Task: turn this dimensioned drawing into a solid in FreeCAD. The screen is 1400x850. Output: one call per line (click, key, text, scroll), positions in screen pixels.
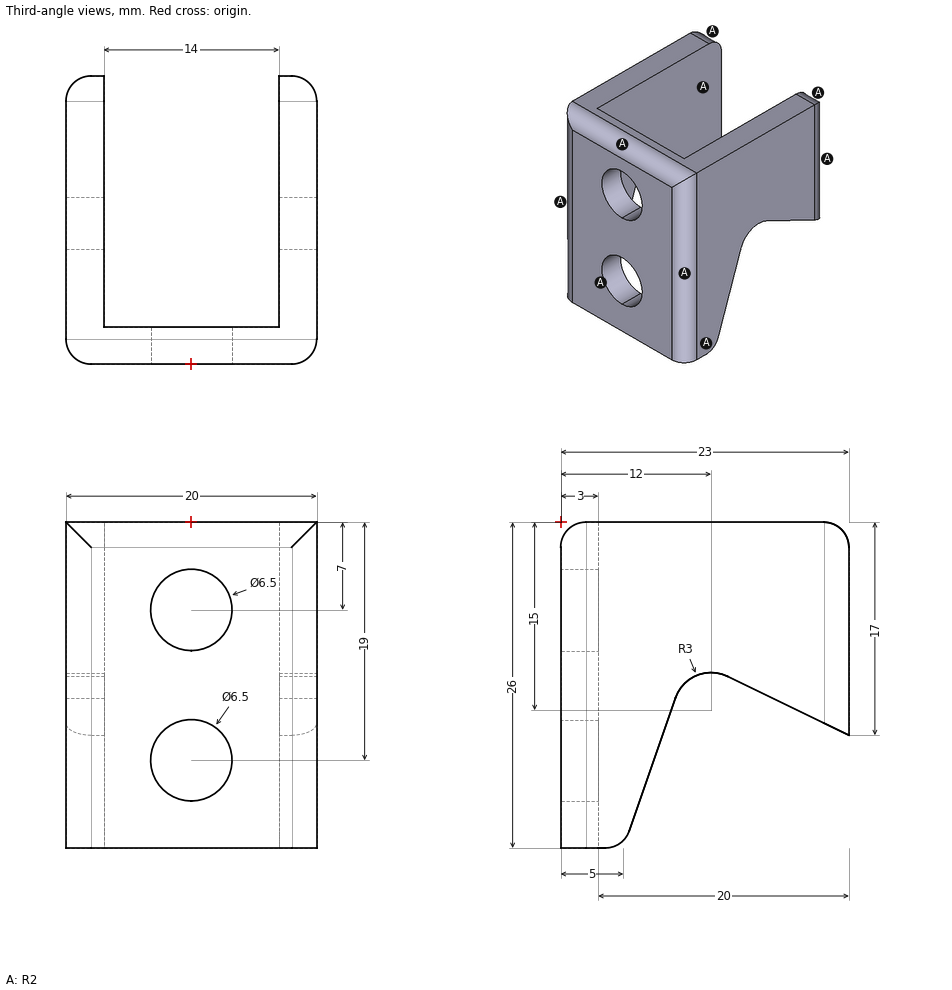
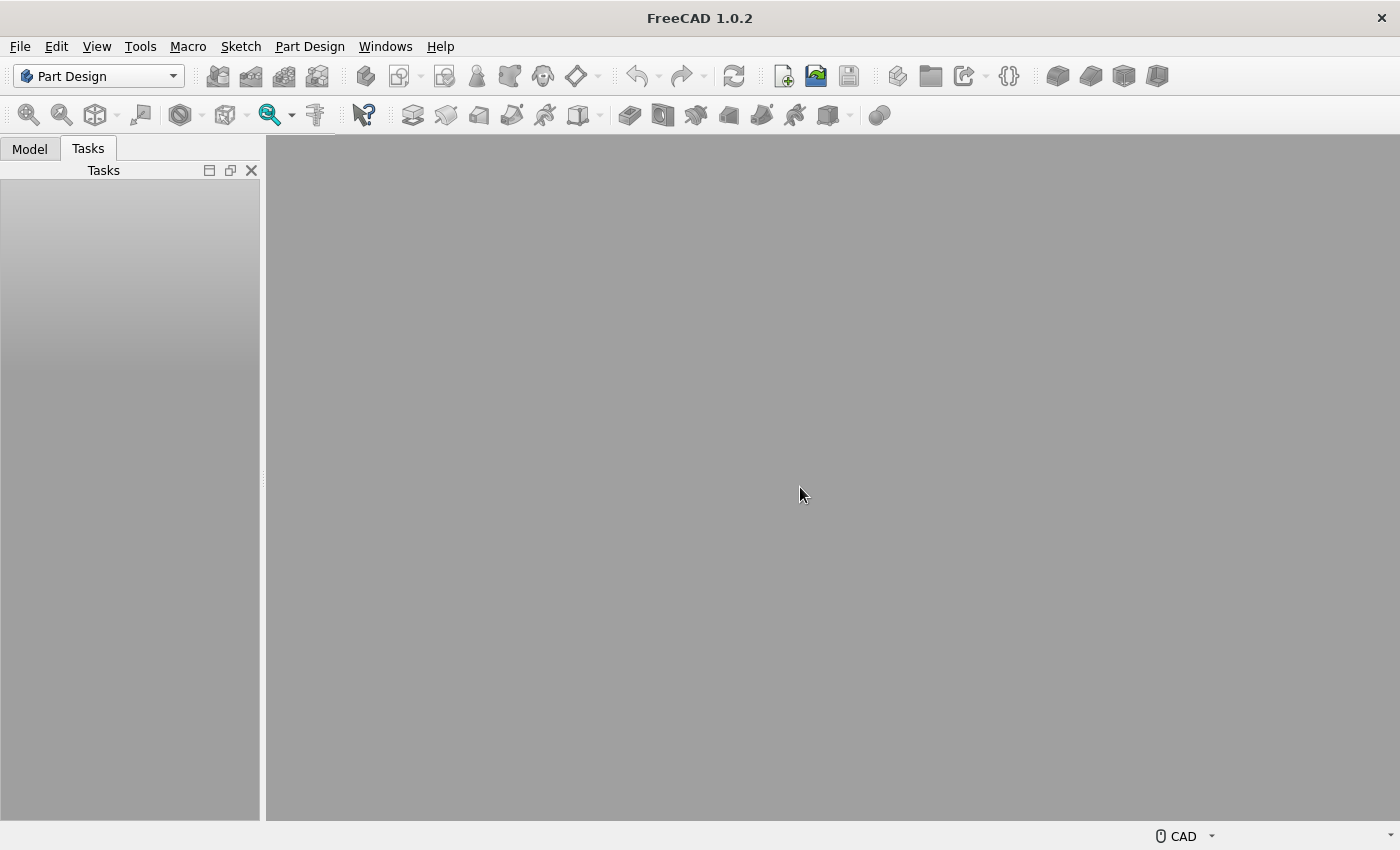
click(783, 76)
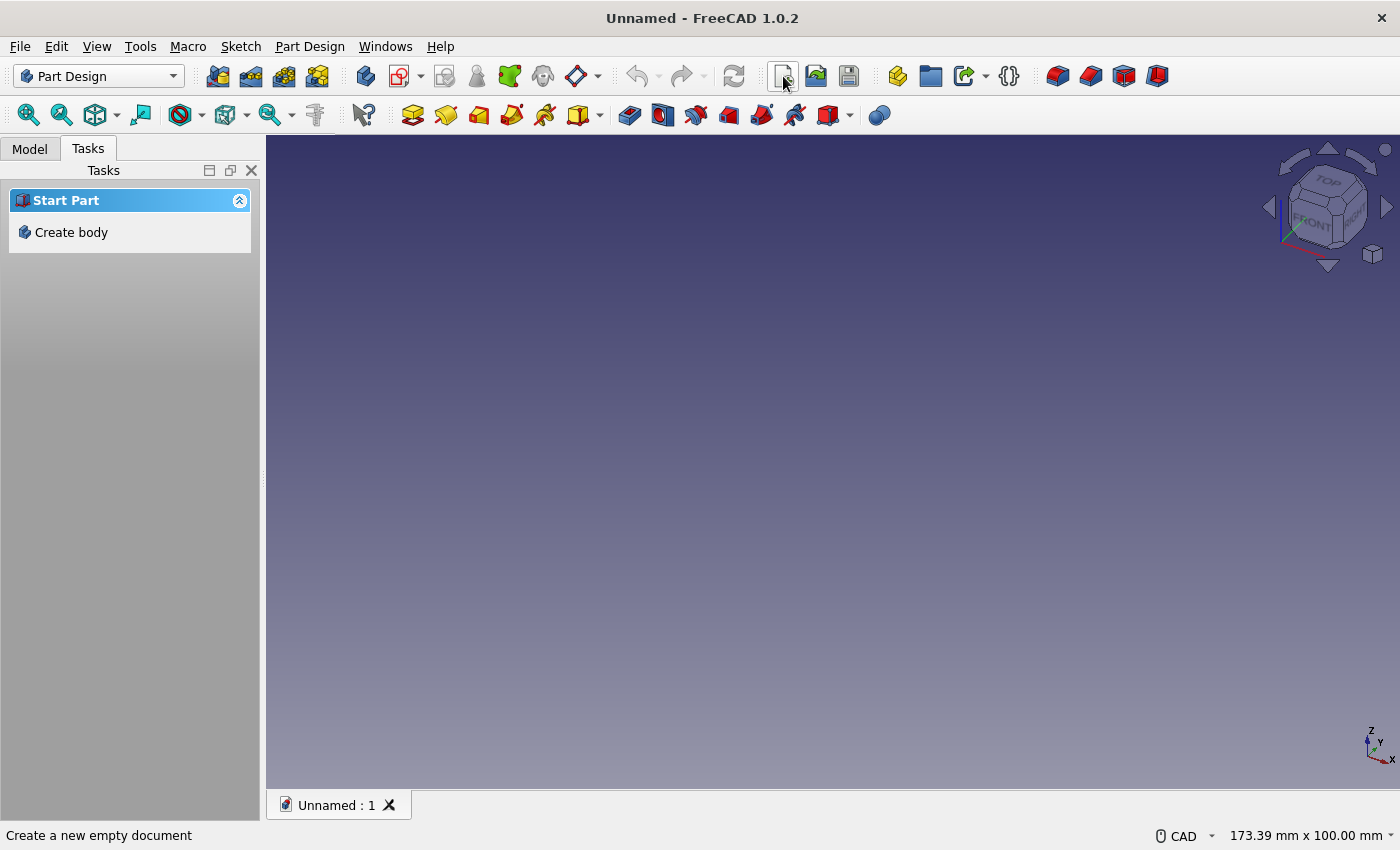
click(398, 76)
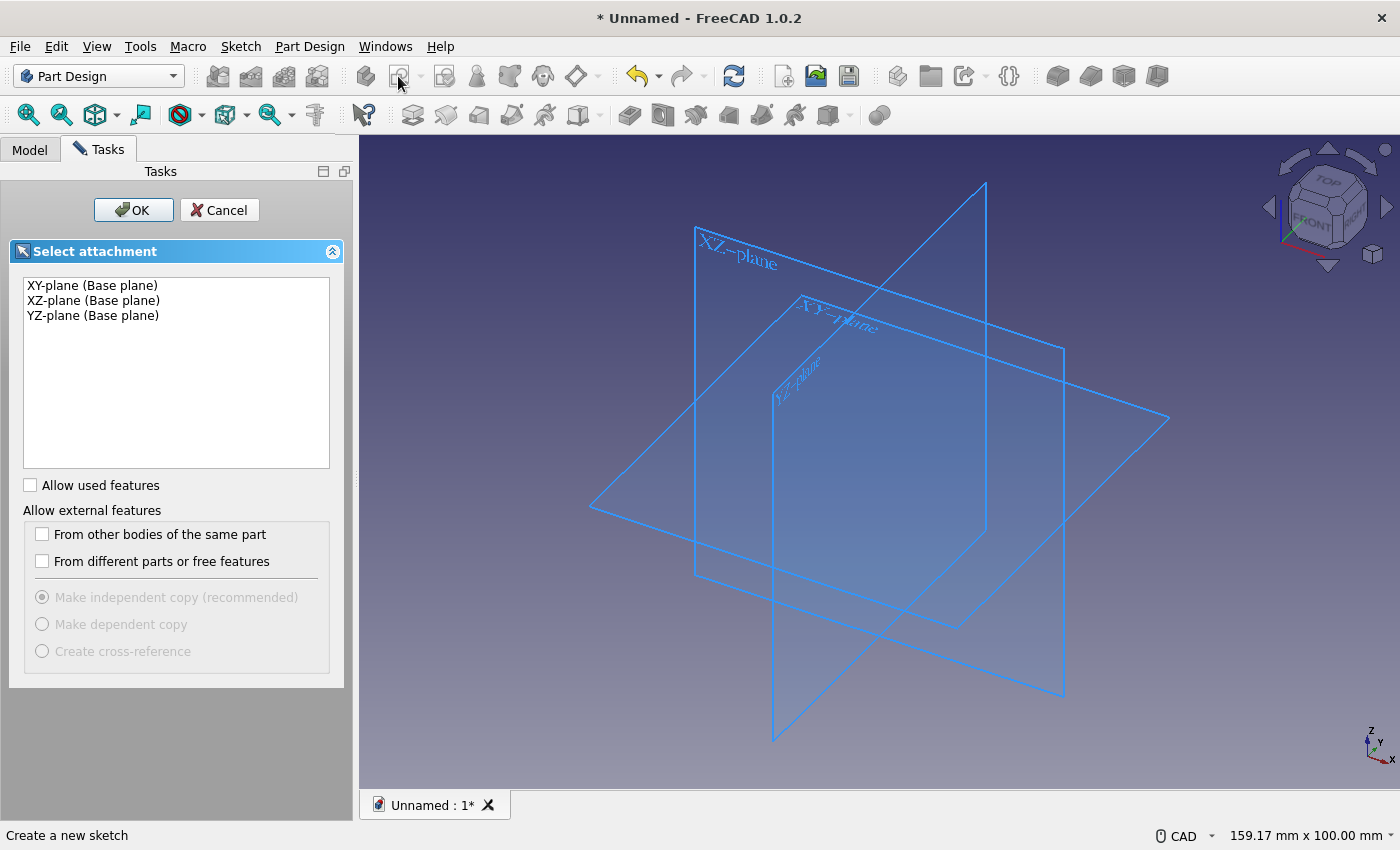
click(84, 316)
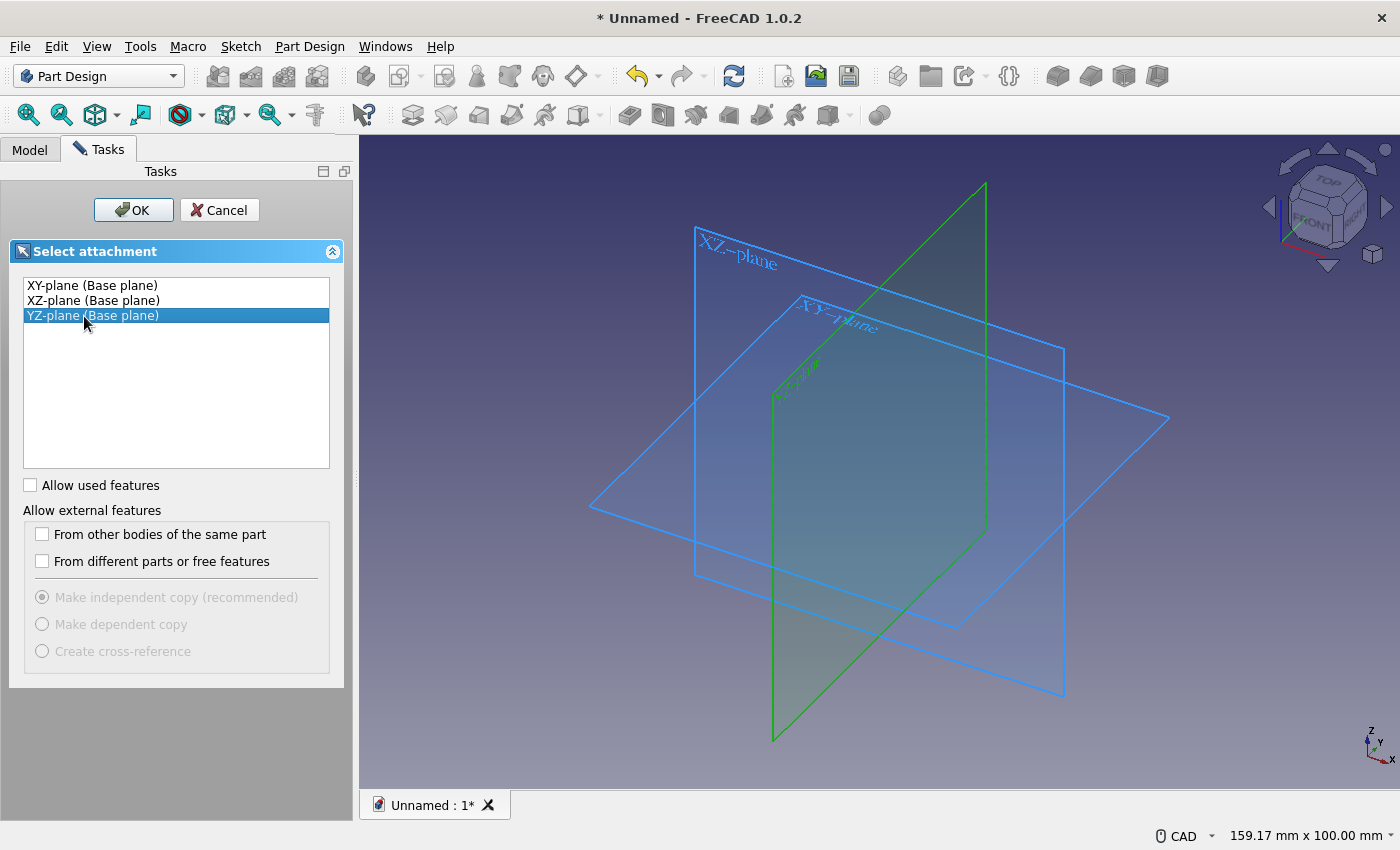
click(134, 210)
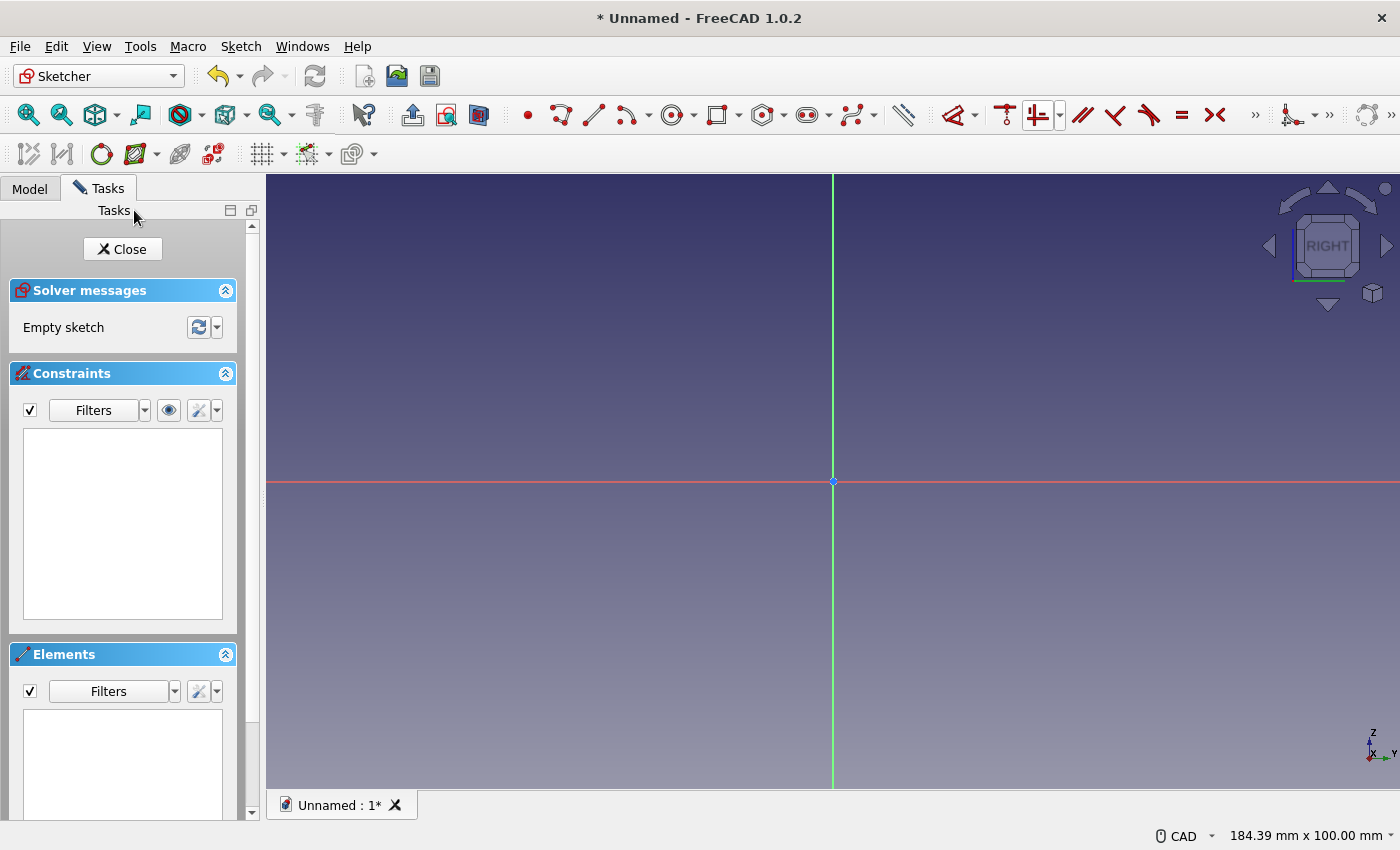
scroll(985, 608, up, 5)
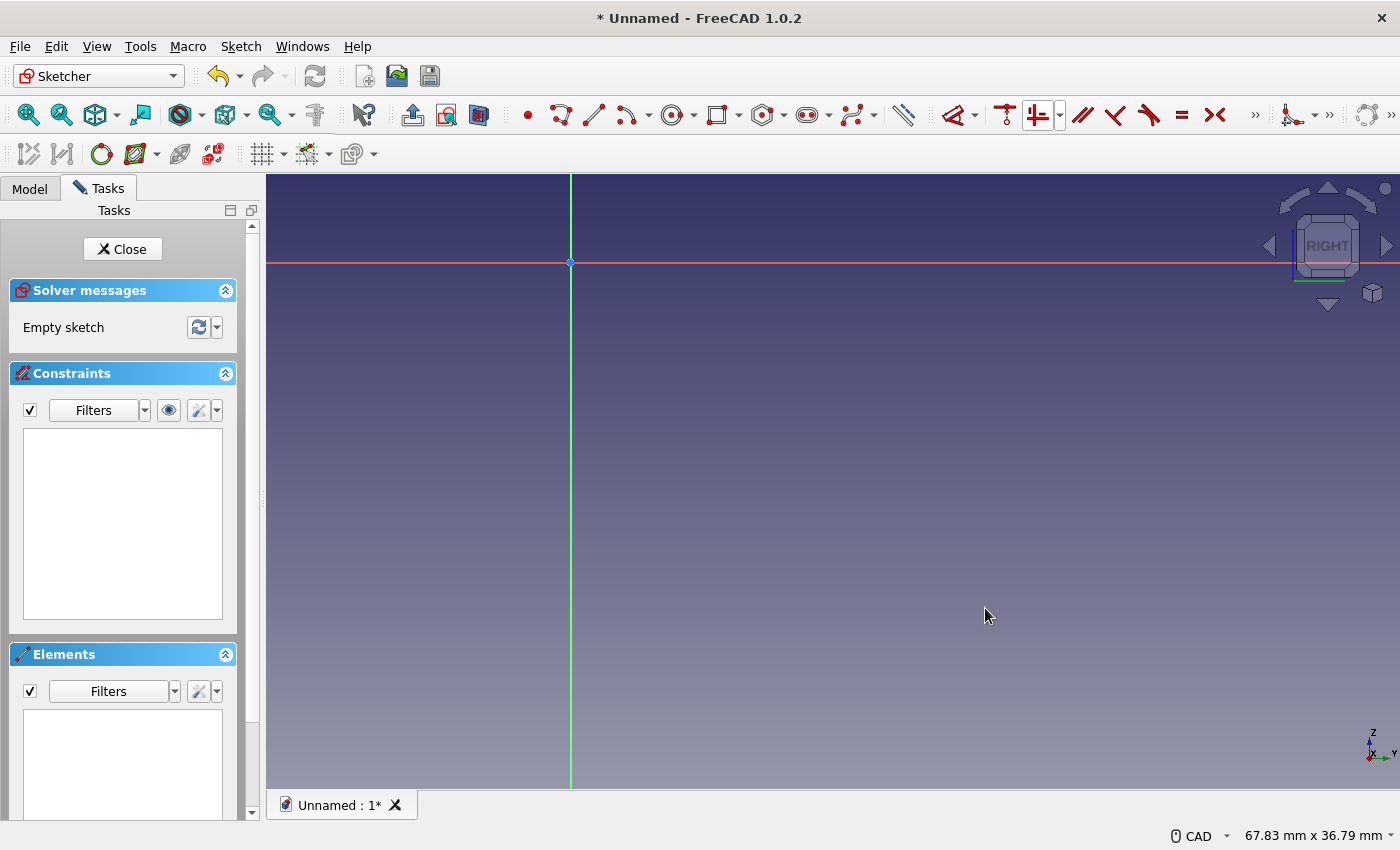
click(561, 116)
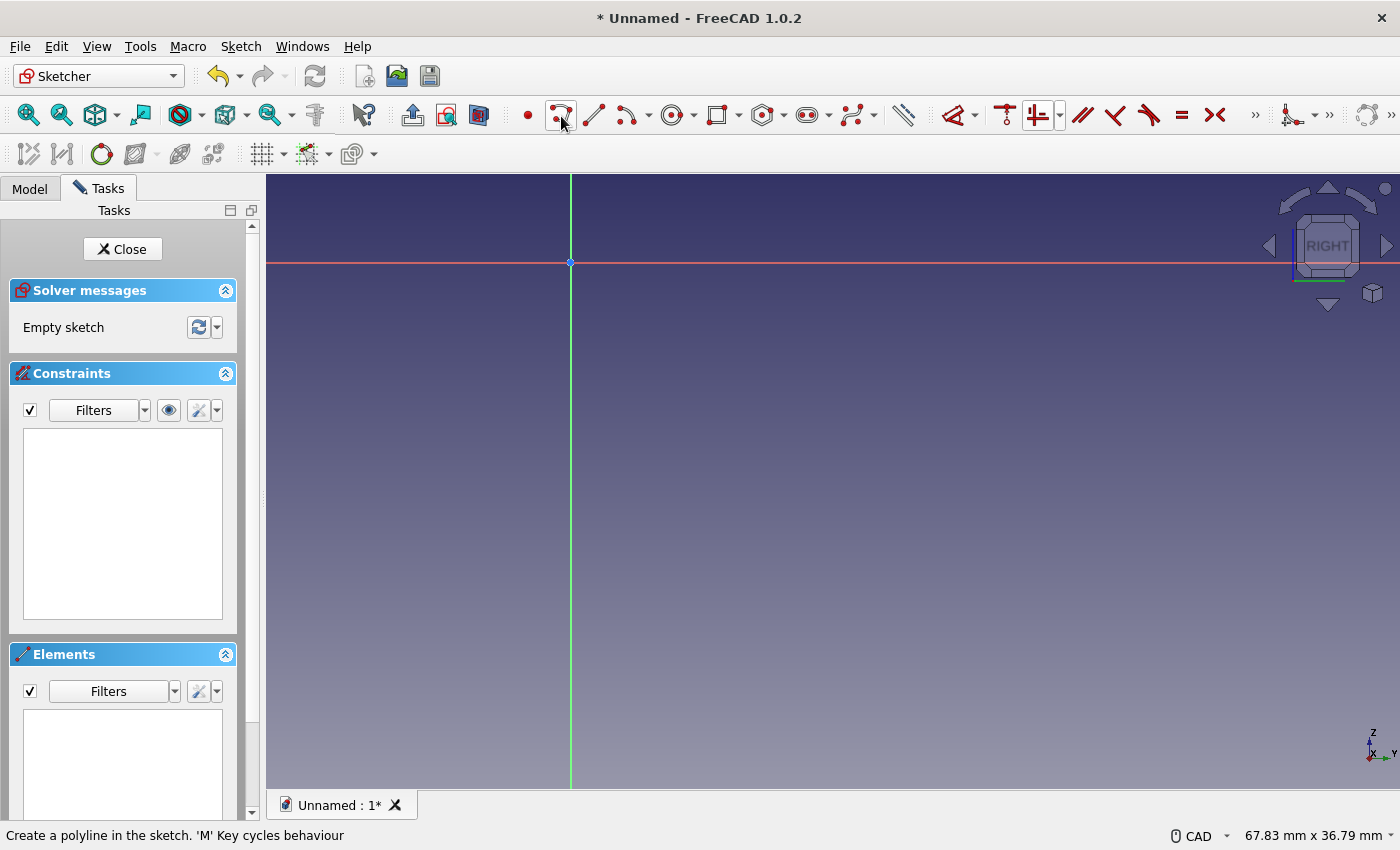
click(793, 469)
click(955, 547)
click(955, 263)
click(571, 263)
click(580, 698)
click(654, 698)
click(724, 497)
right_click(724, 497)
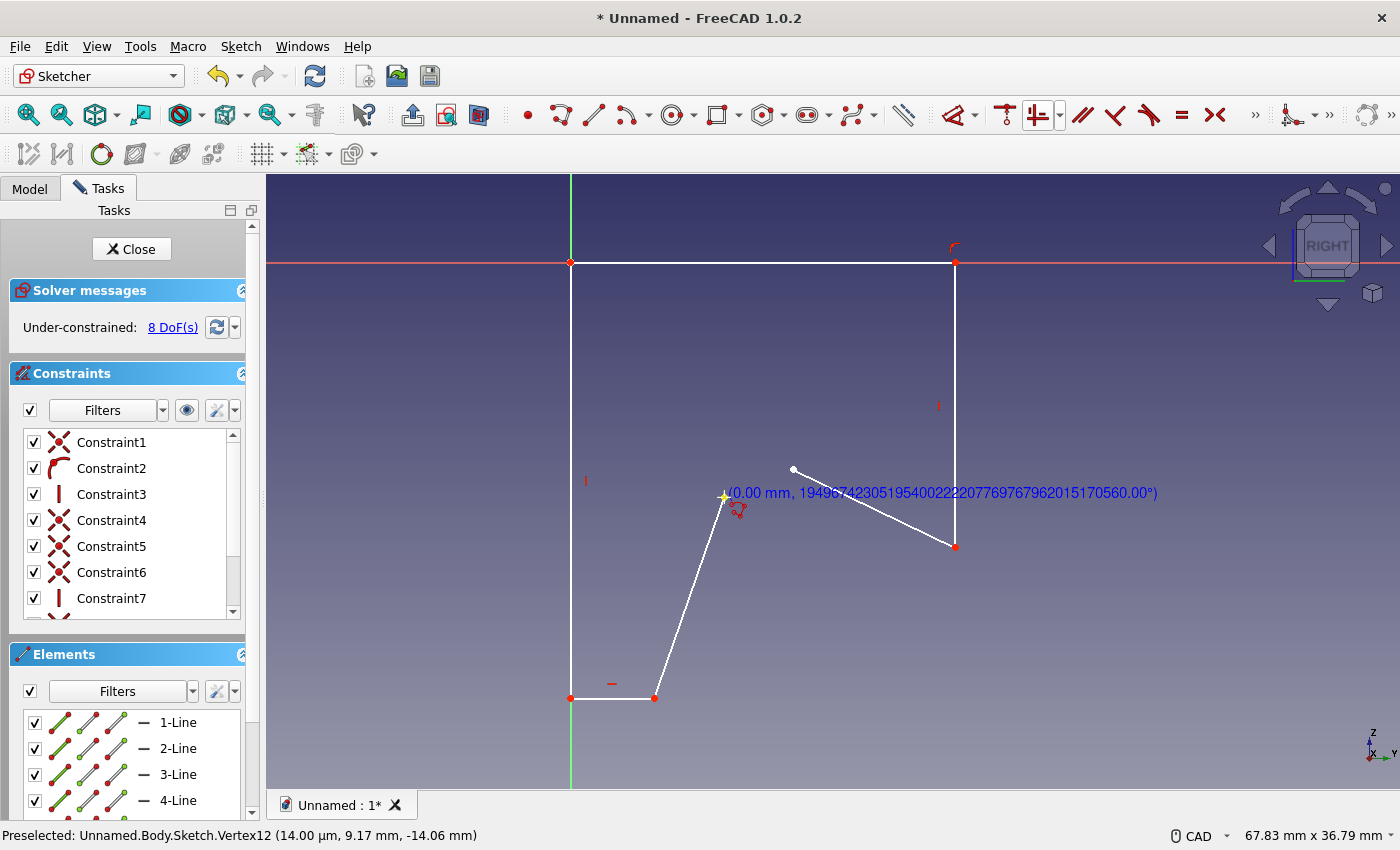
key(g)
key(3)
key(a)